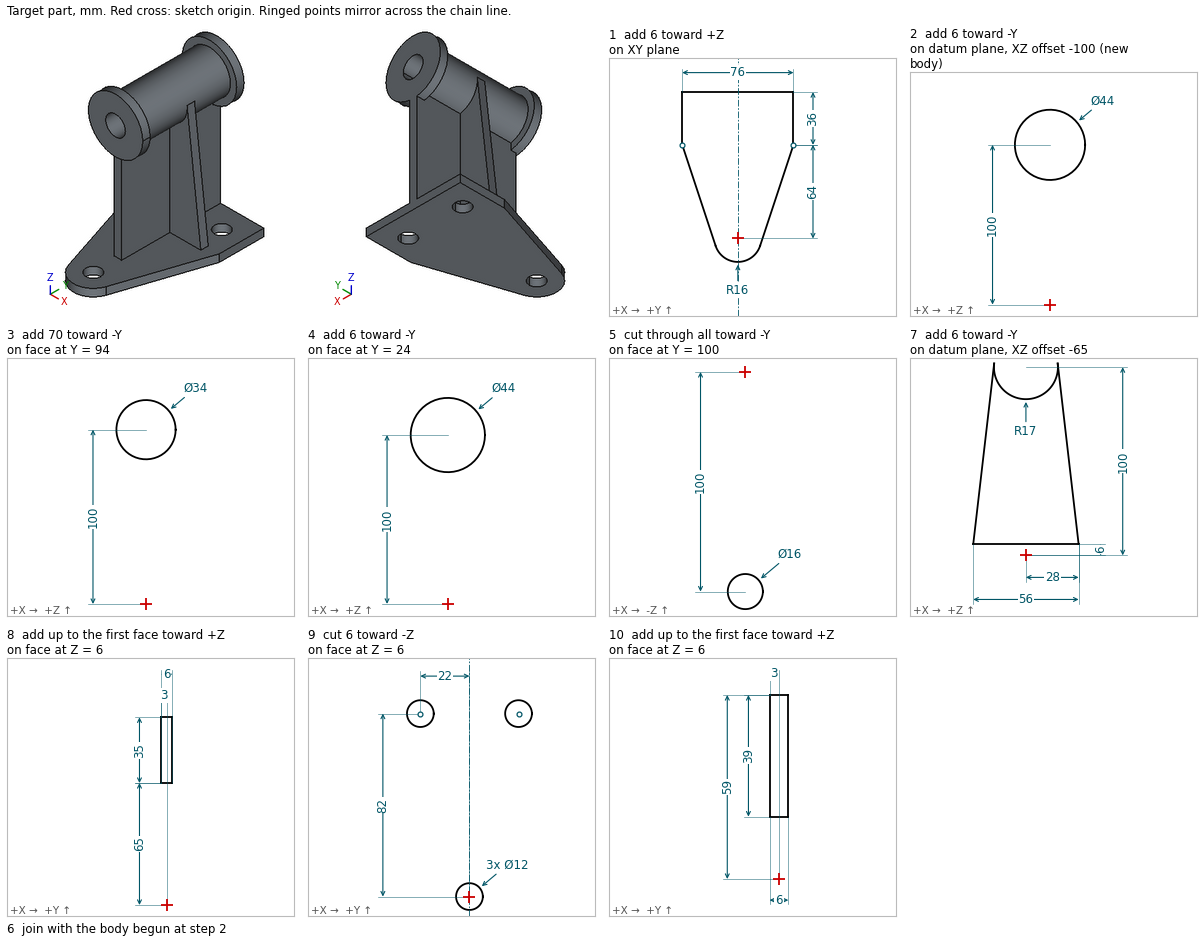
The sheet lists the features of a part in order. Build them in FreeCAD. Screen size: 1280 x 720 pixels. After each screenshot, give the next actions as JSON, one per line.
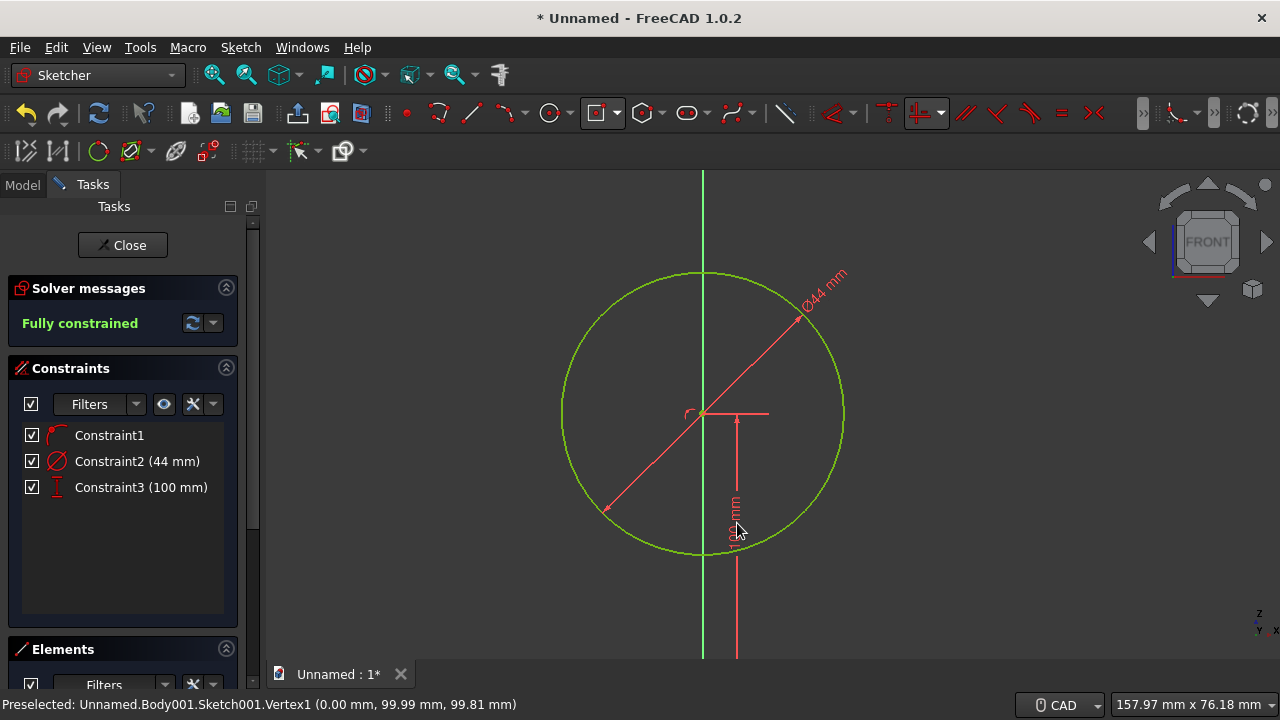
{"action": "left_click", "coordinate": [123, 245]}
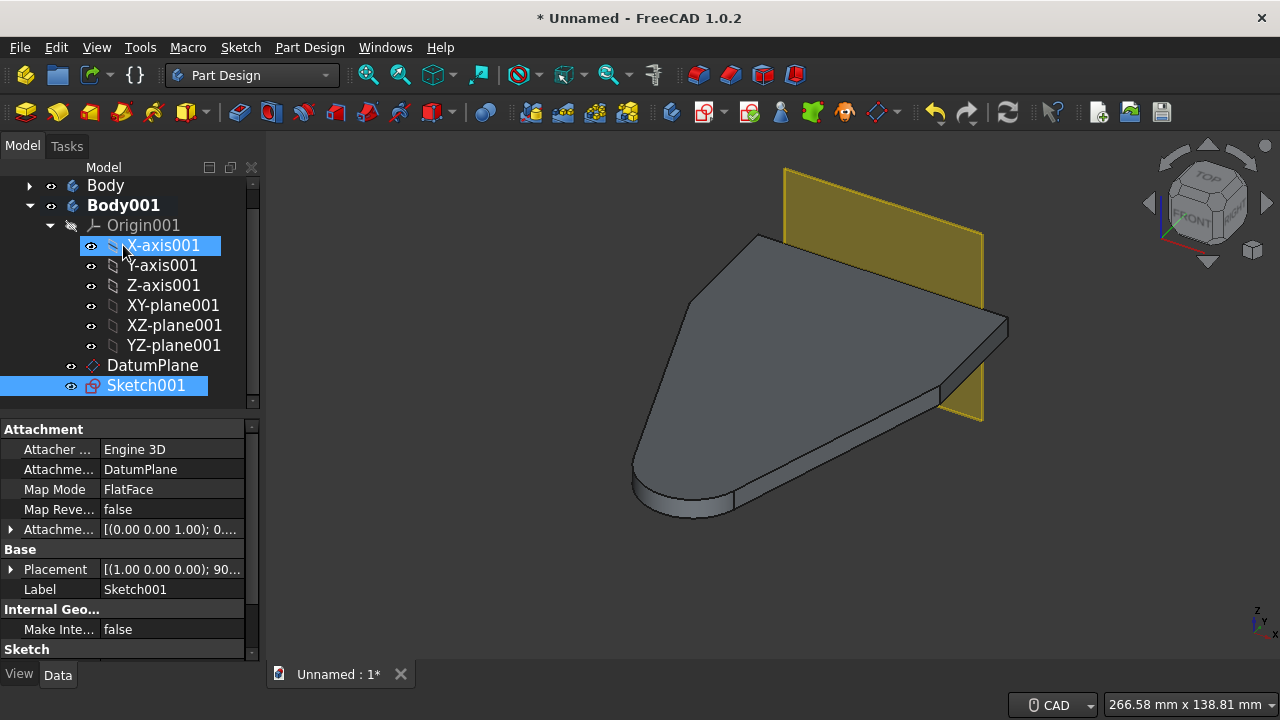
{"action": "left_click", "coordinate": [26, 112]}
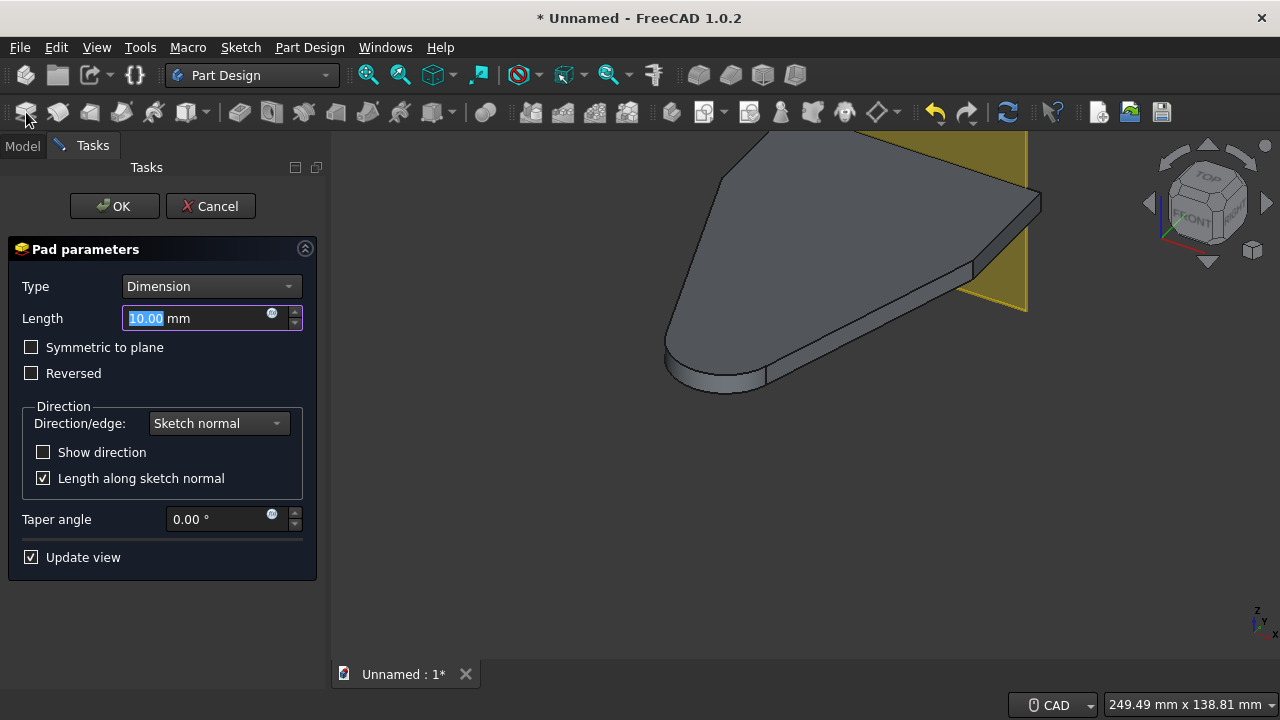
{"action": "type", "text": "6"}
{"action": "key", "text": "Tab"}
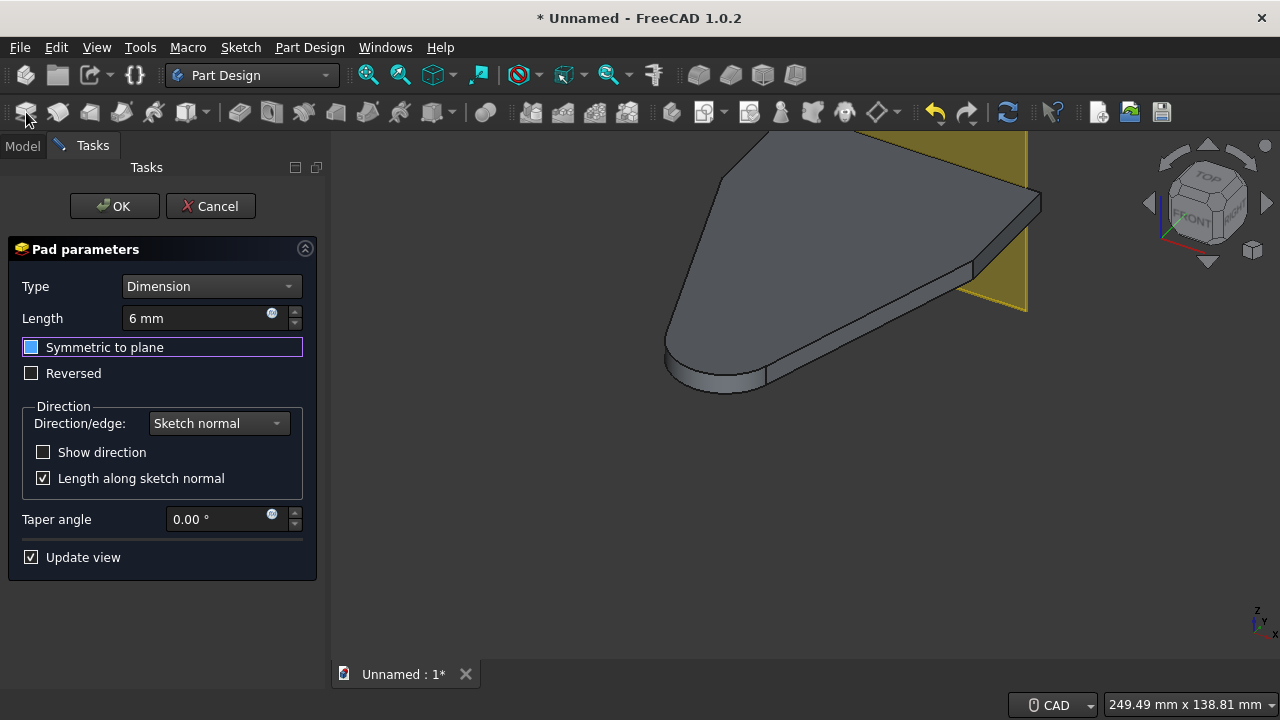
{"action": "left_click", "coordinate": [115, 206]}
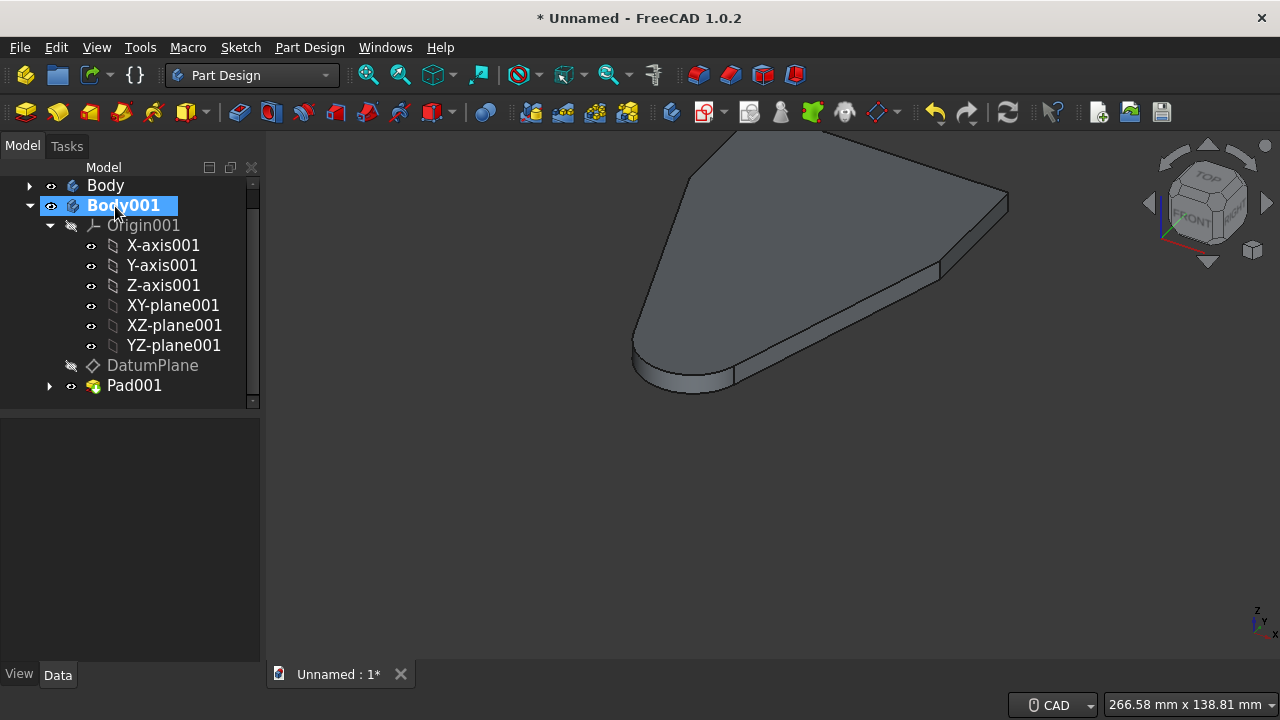
{"action": "key", "text": "v f"}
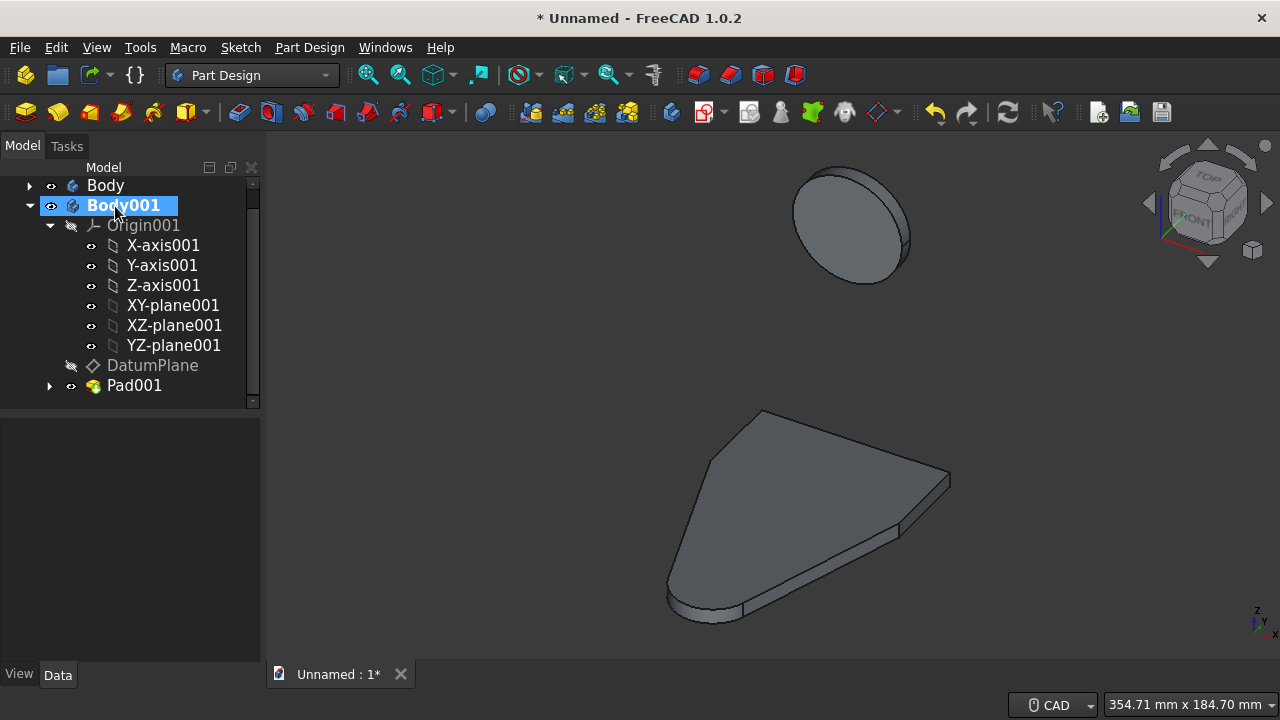
{"action": "left_click", "coordinate": [847, 229]}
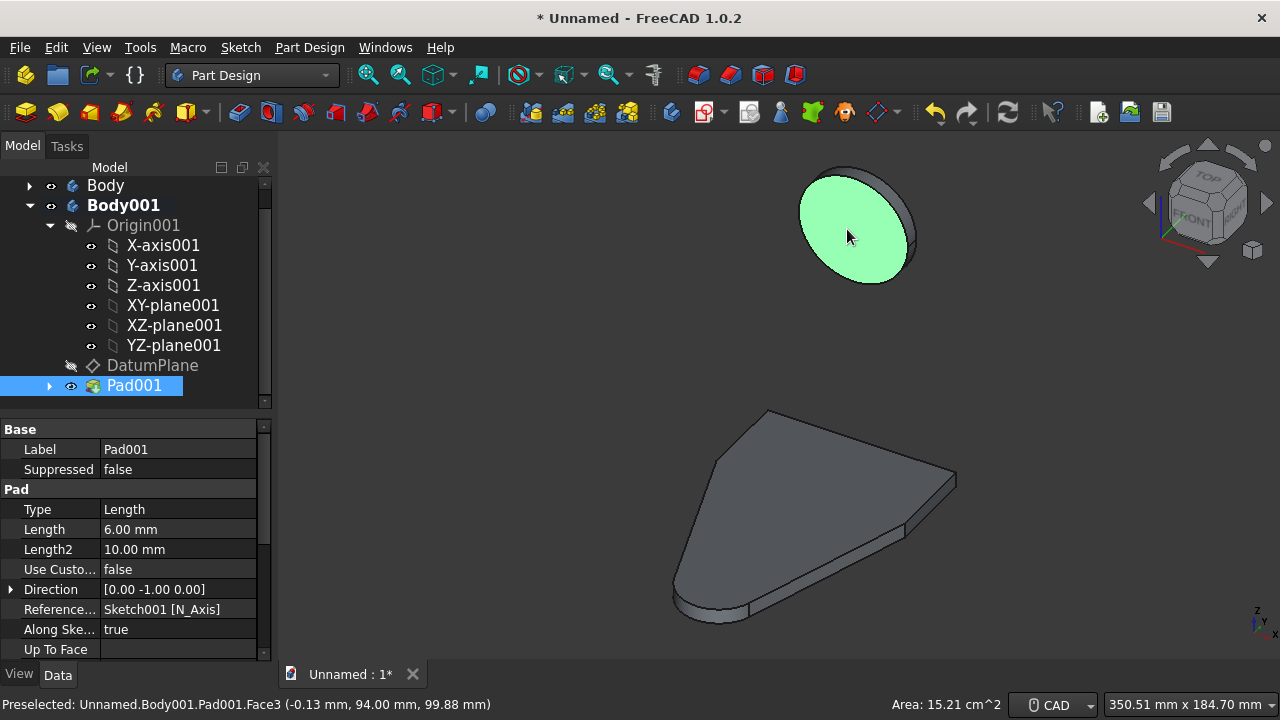
{"action": "left_click", "coordinate": [704, 112]}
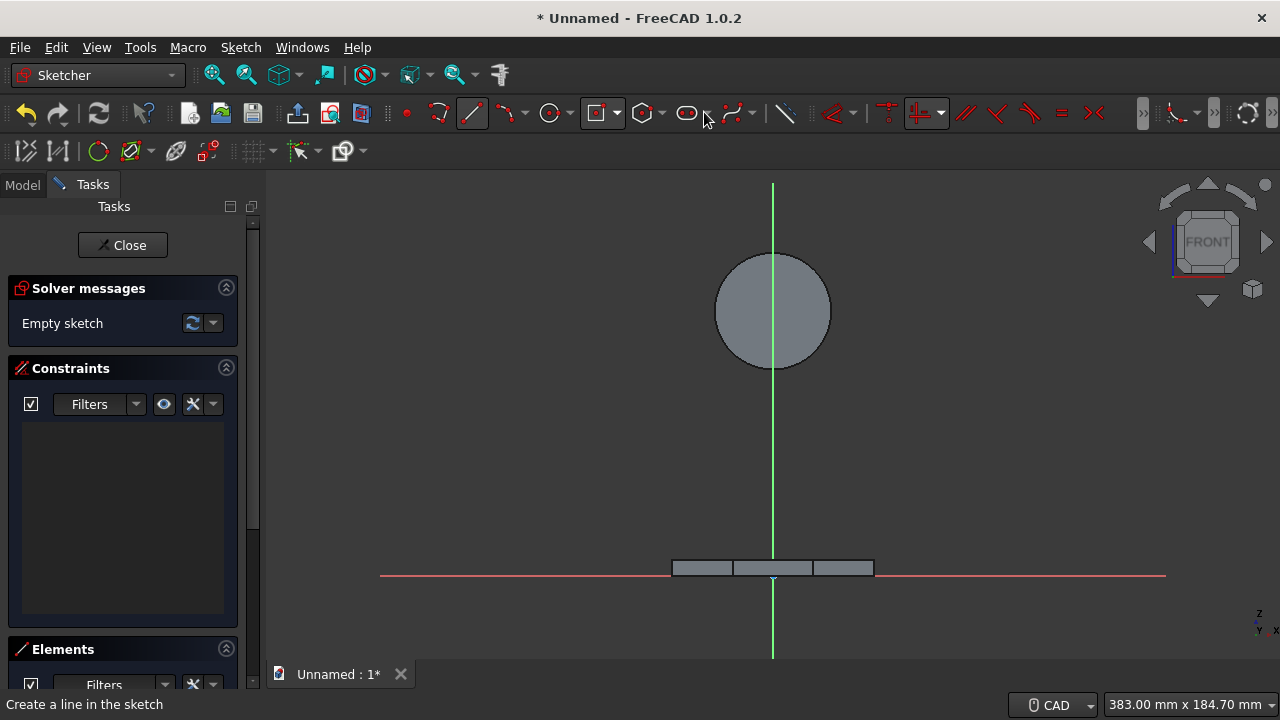
{"action": "scroll", "coordinate": [803, 267], "scroll_direction": "up", "scroll_amount": 6}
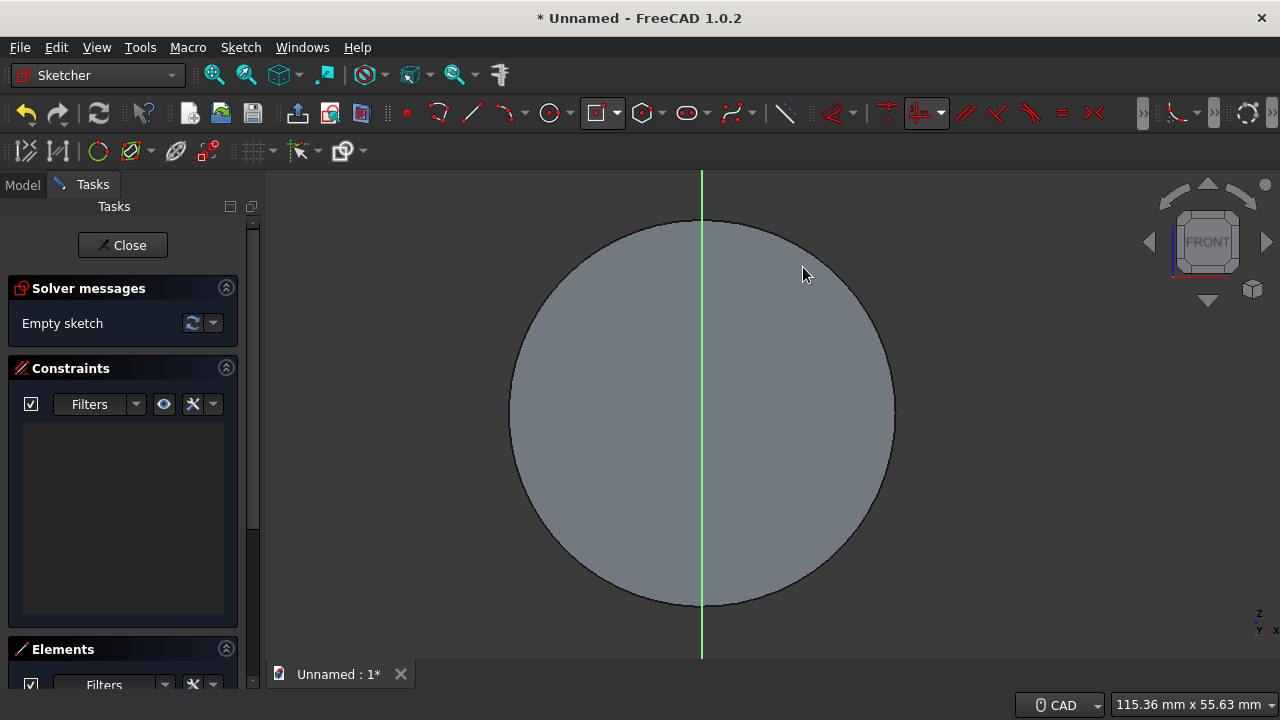
{"action": "key", "text": "g c"}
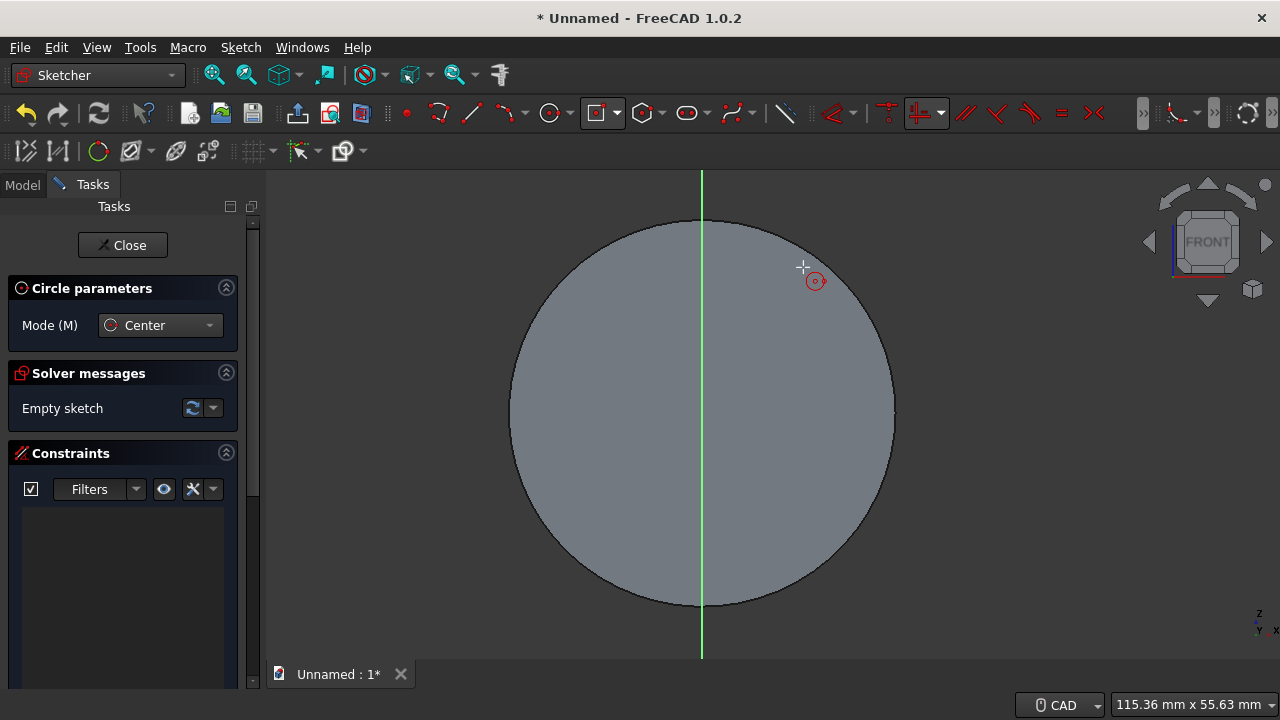
{"action": "left_click", "coordinate": [702, 413]}
{"action": "left_click", "coordinate": [808, 308]}
{"action": "key", "text": "Escape"}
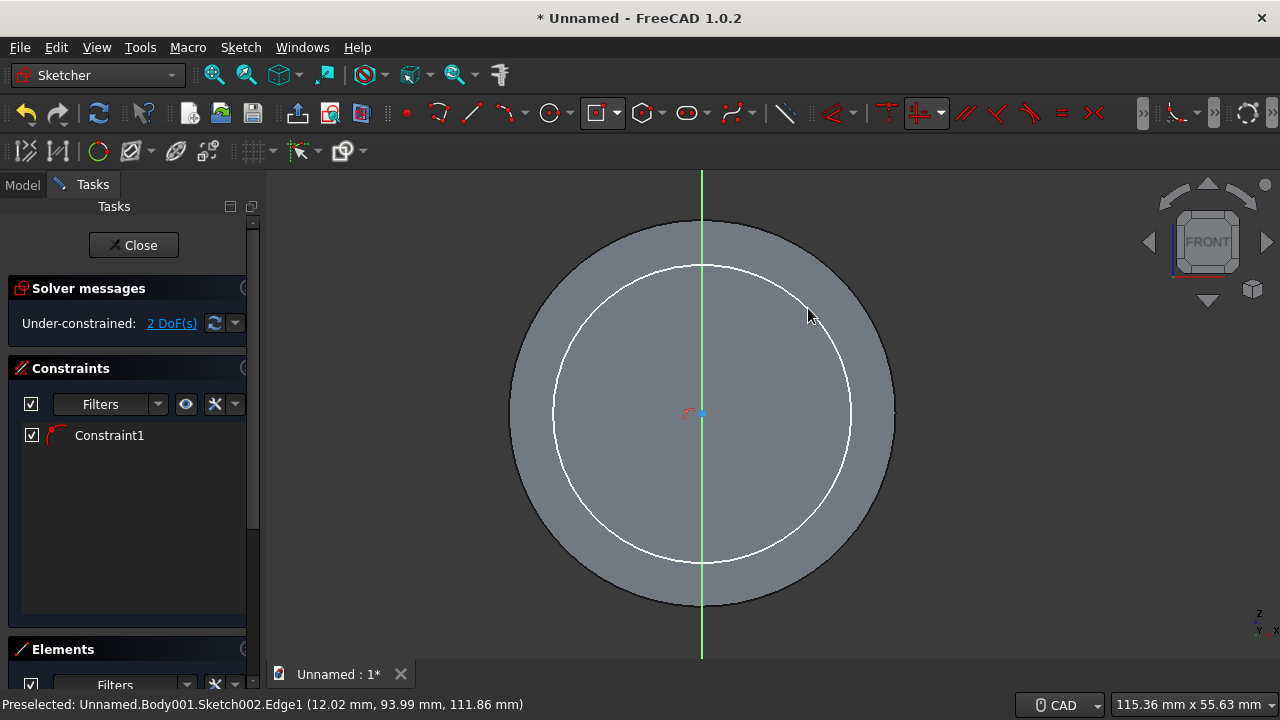
{"action": "key", "text": "d"}